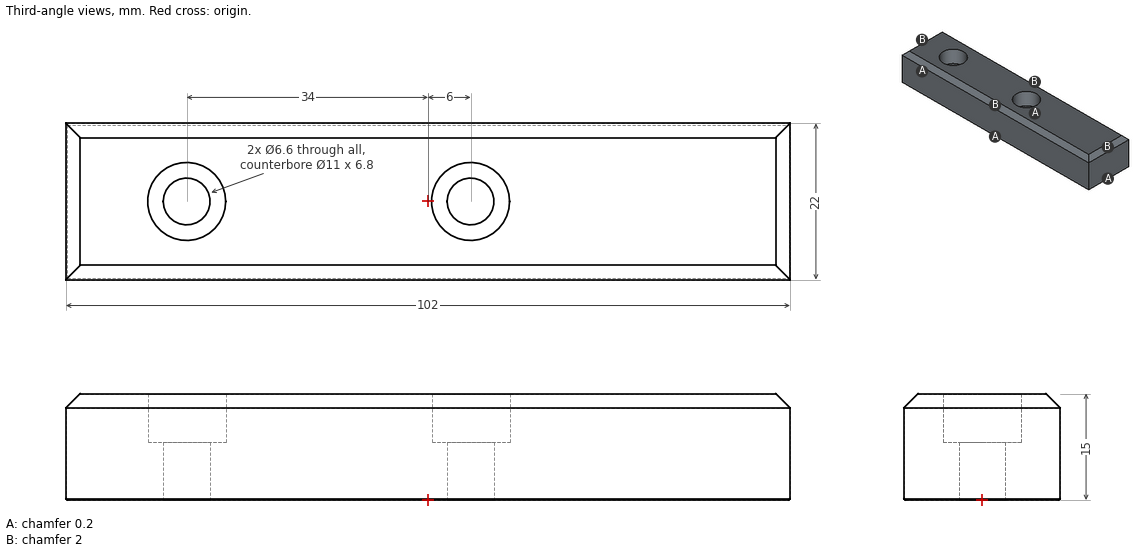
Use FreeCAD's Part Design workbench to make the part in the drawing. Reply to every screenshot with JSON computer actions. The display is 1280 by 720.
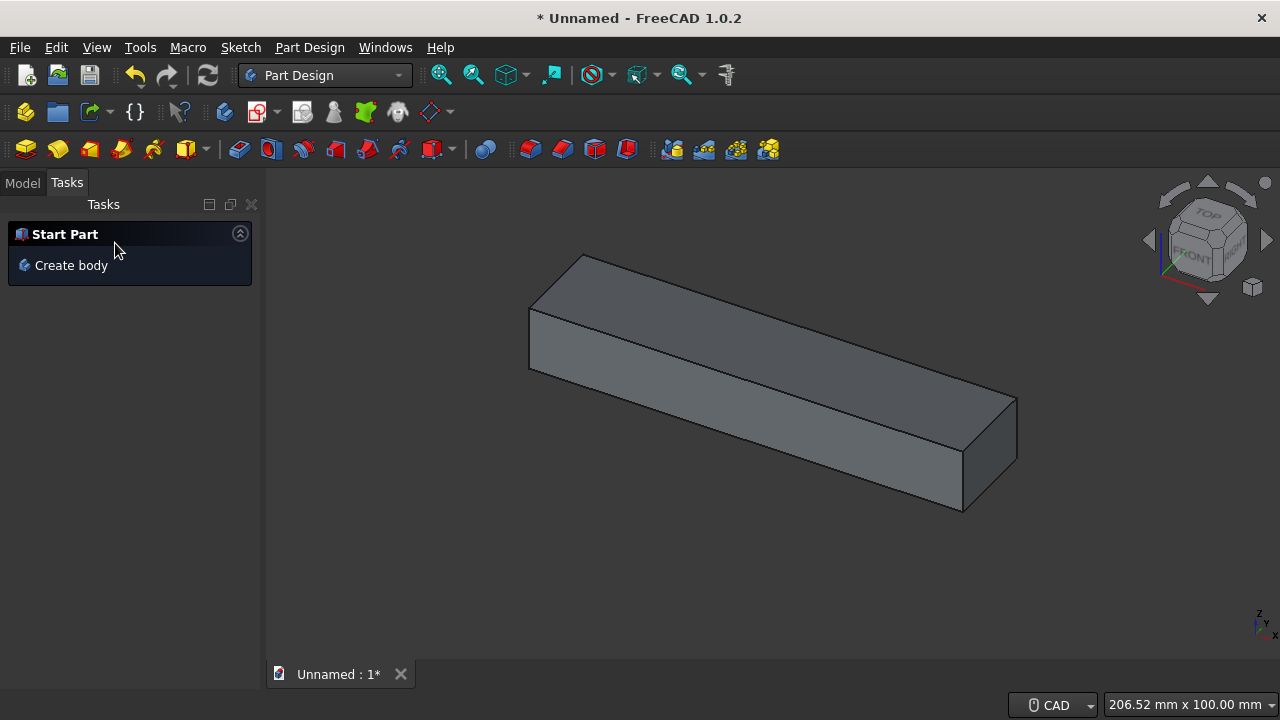
{"action": "left_click", "coordinate": [897, 393]}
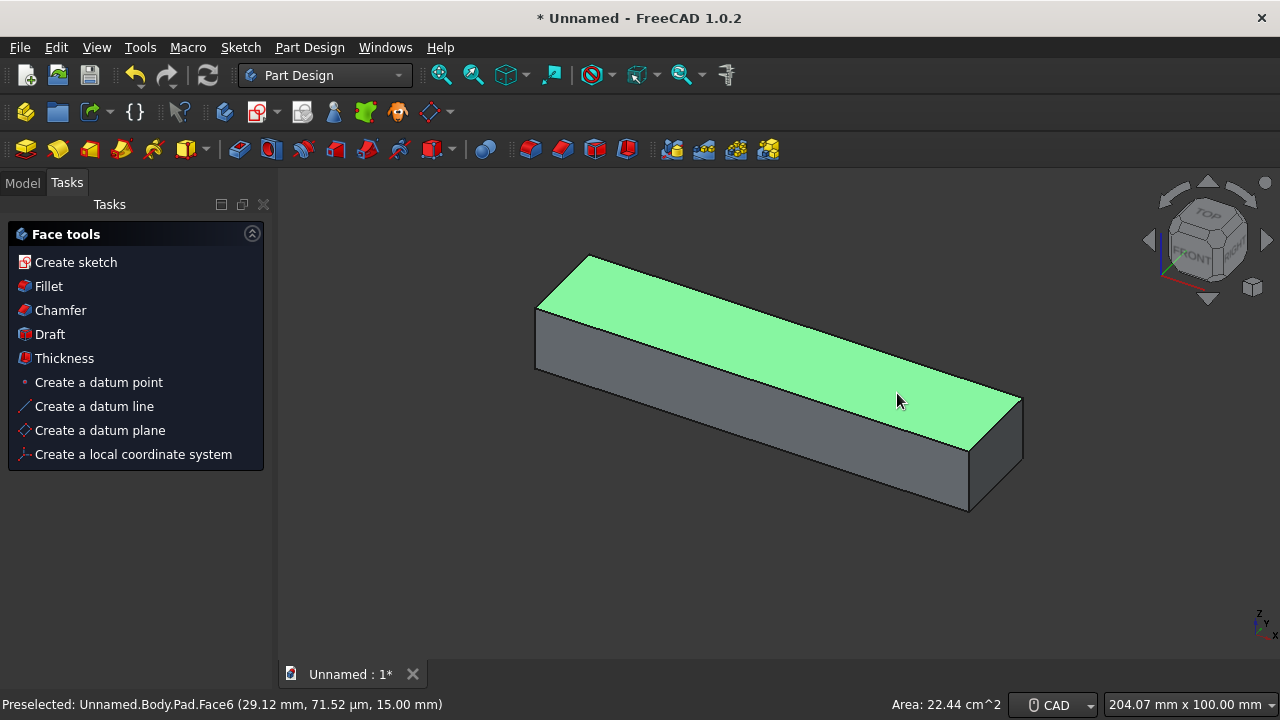
{"action": "left_click", "coordinate": [258, 112]}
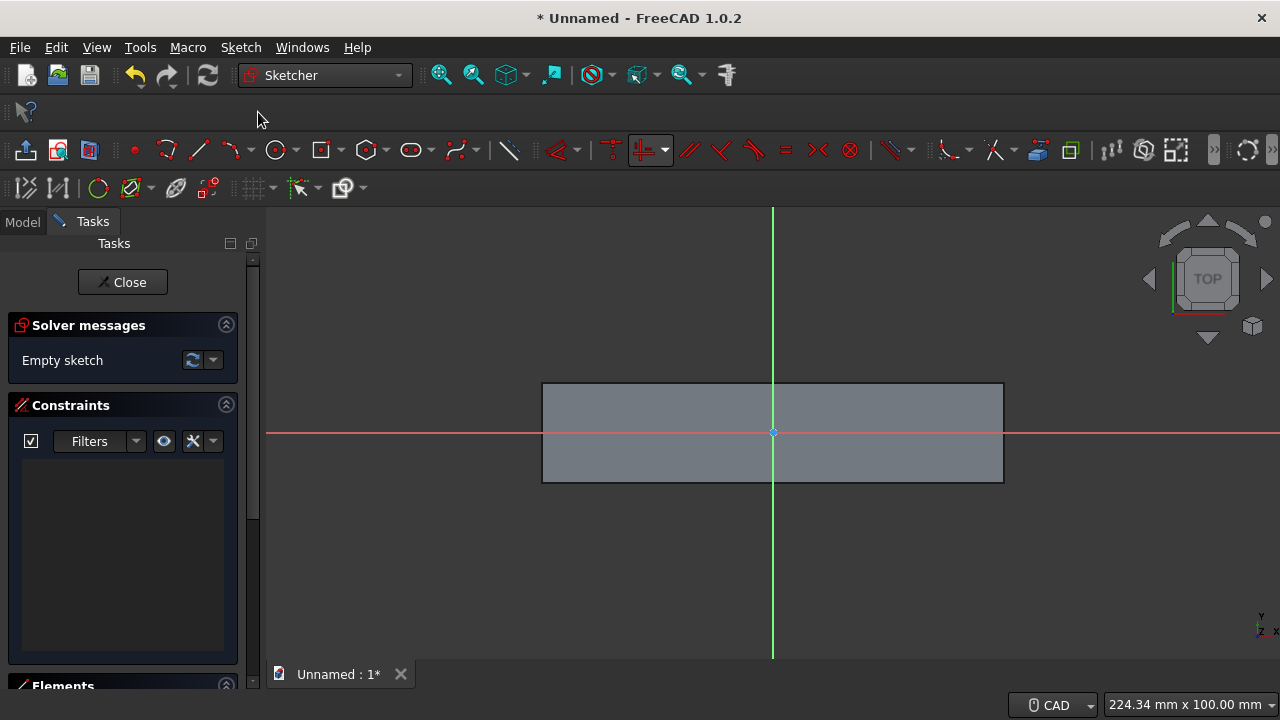
{"action": "scroll", "coordinate": [713, 433], "scroll_direction": "up", "scroll_amount": 5}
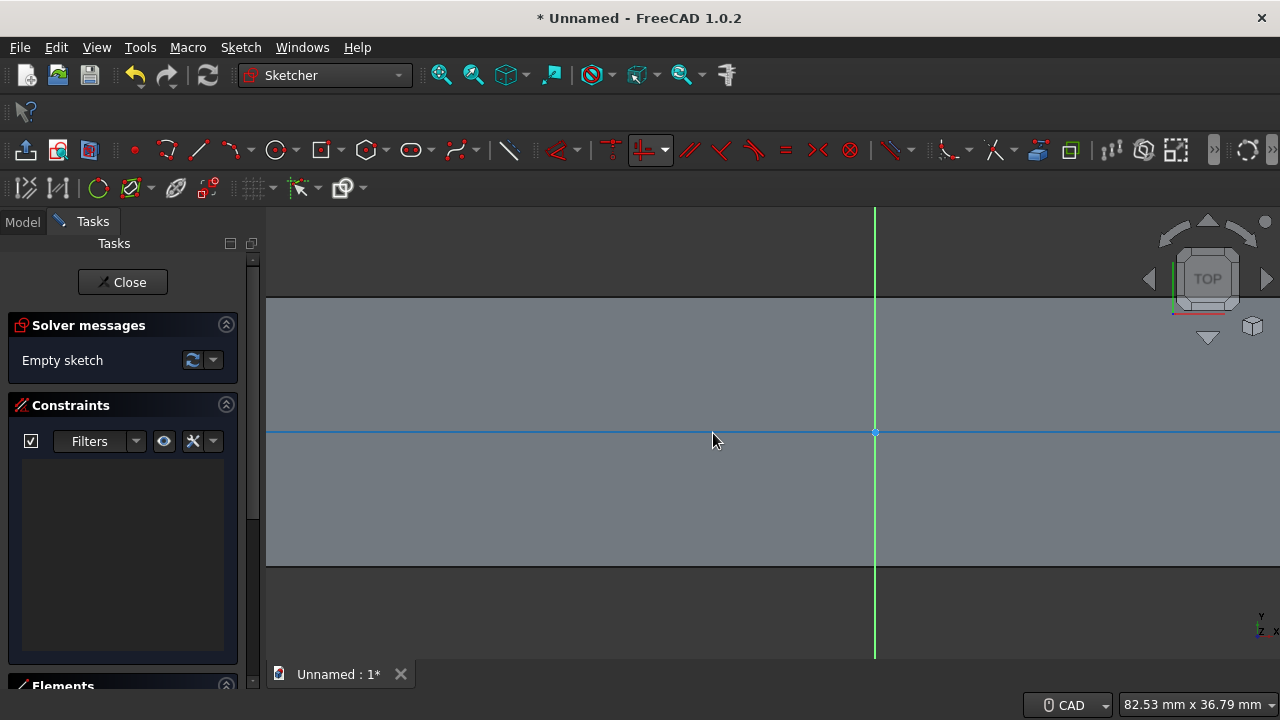
{"action": "left_click", "coordinate": [276, 150]}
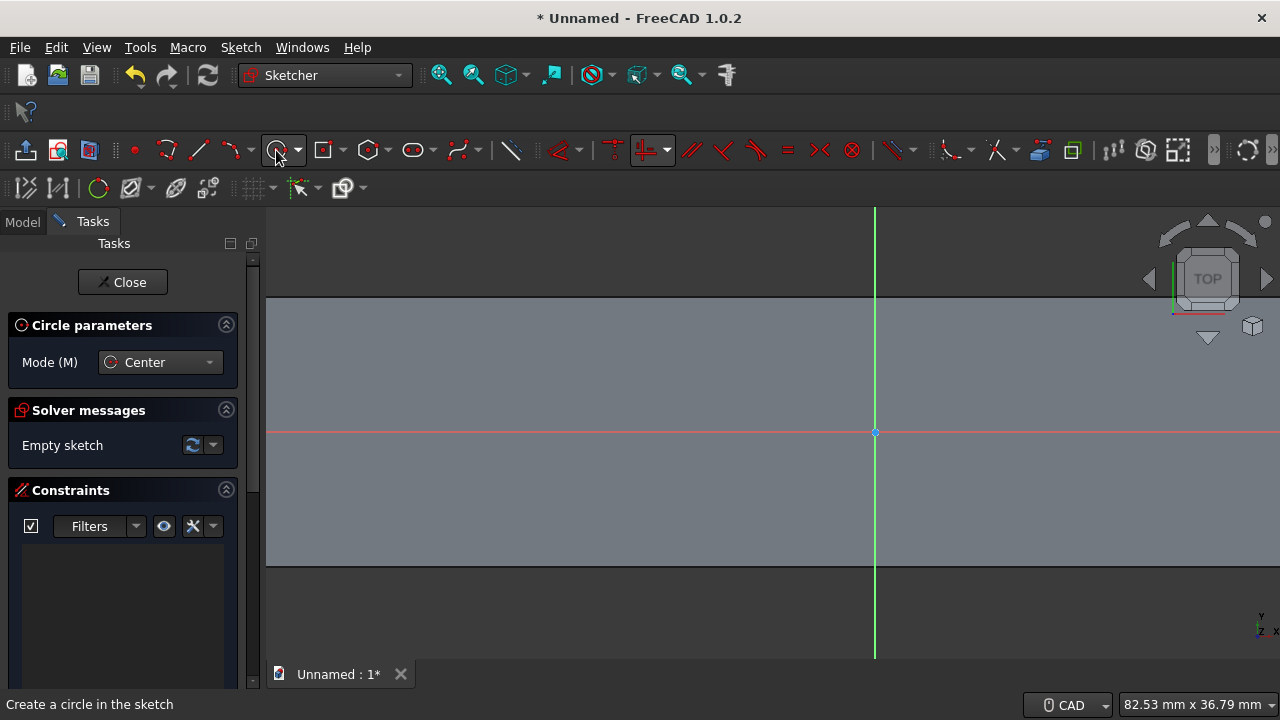
{"action": "left_click", "coordinate": [458, 432]}
{"action": "mouse_move", "coordinate": [486, 403]}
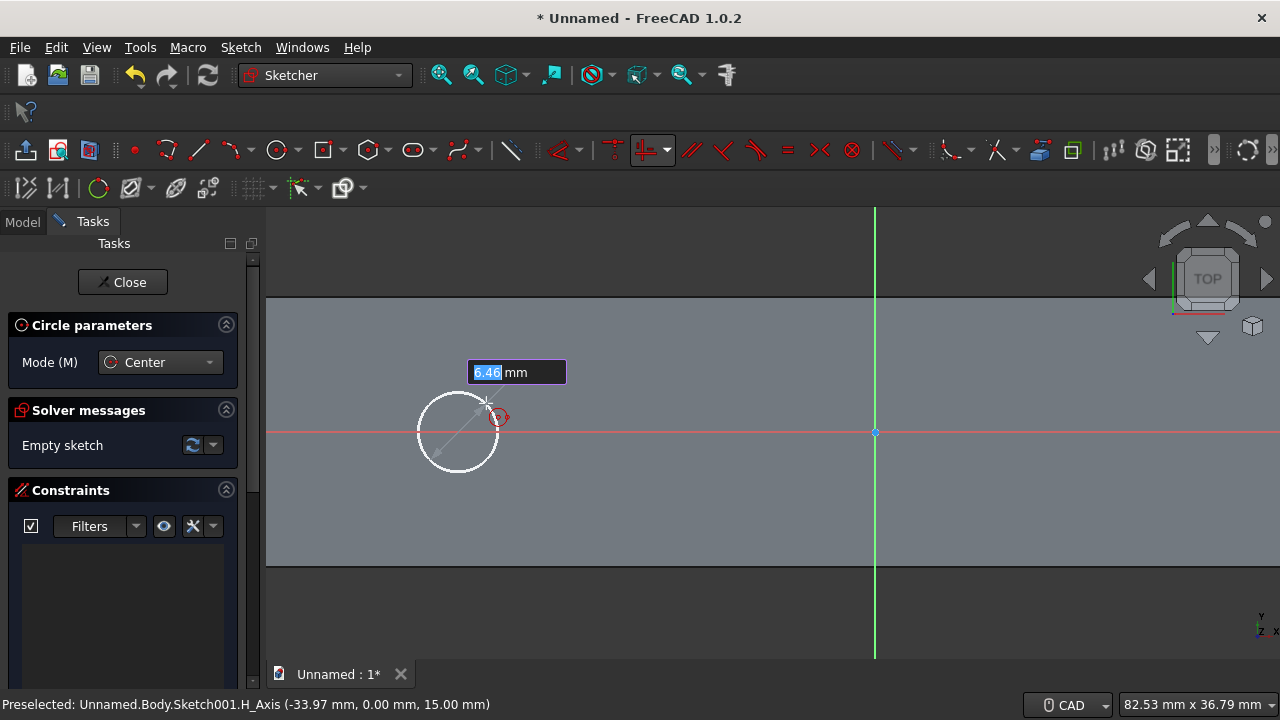
{"action": "type", "text": "6.6"}
{"action": "key", "text": "Return"}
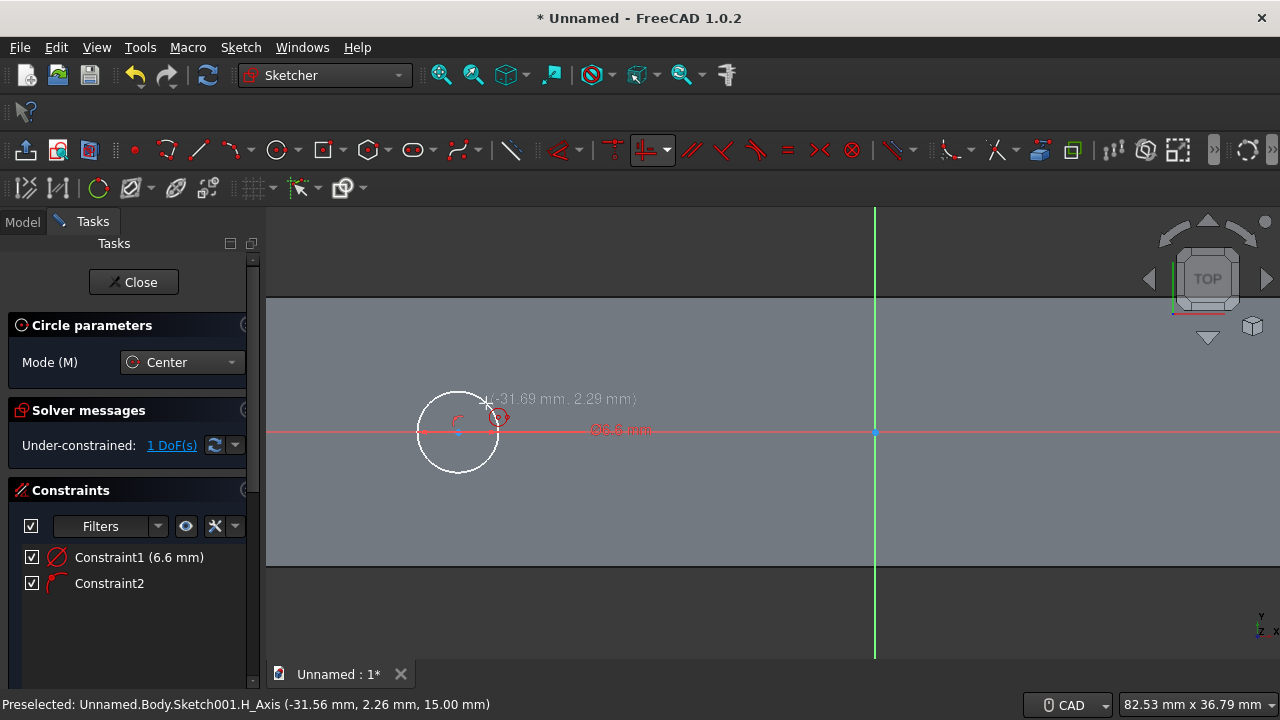
{"action": "left_click", "coordinate": [949, 432]}
{"action": "mouse_move", "coordinate": [978, 403]}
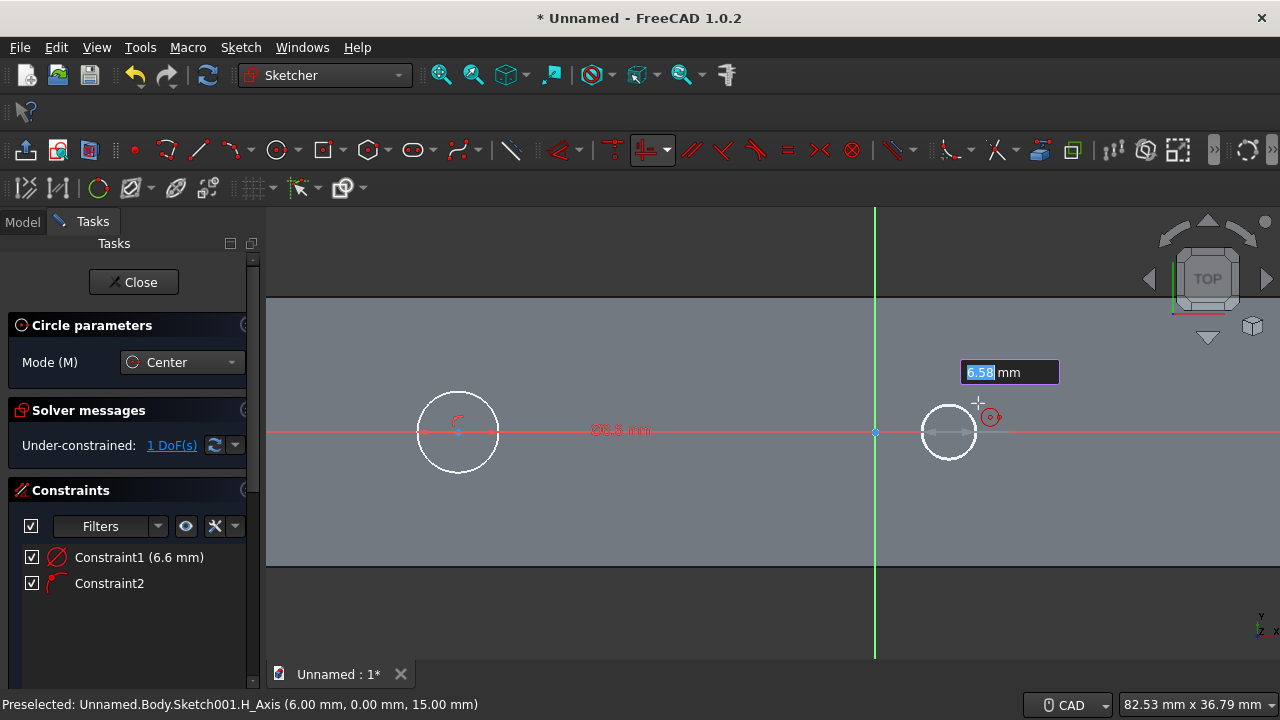
{"action": "type", "text": "6.6"}
{"action": "key", "text": "Return"}
{"action": "key", "text": "Escape"}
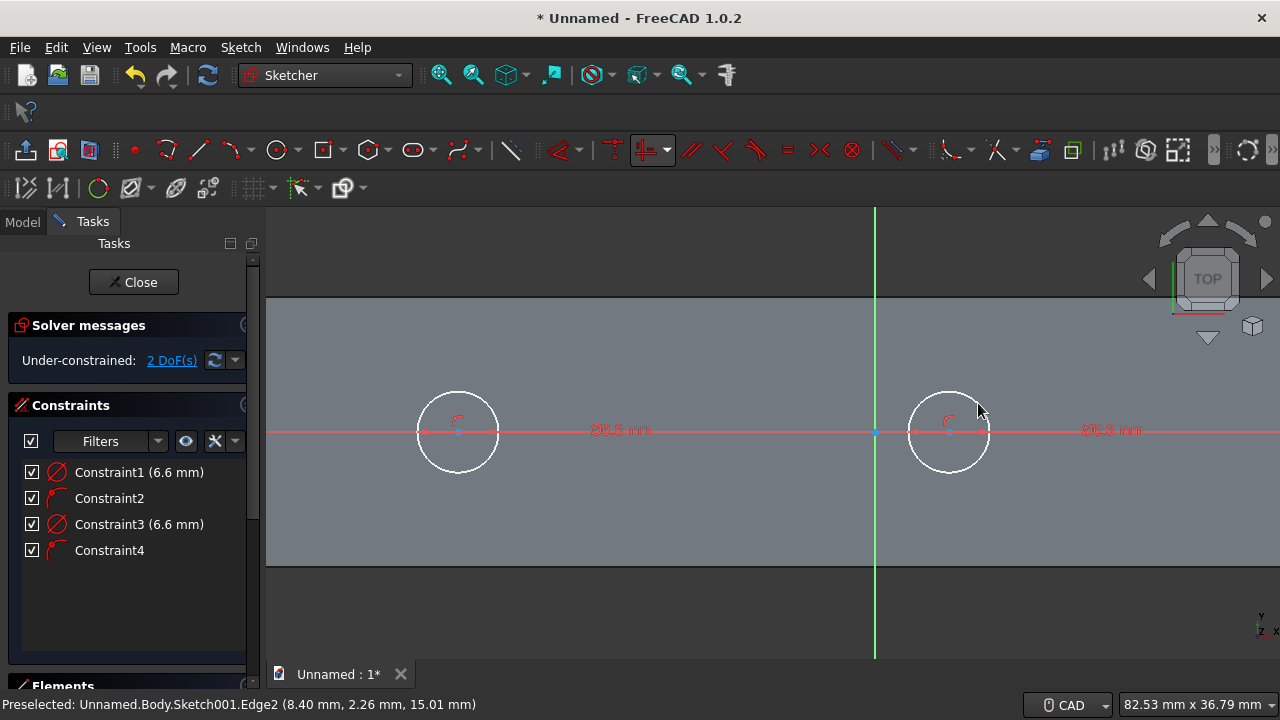
{"action": "left_click", "coordinate": [558, 150]}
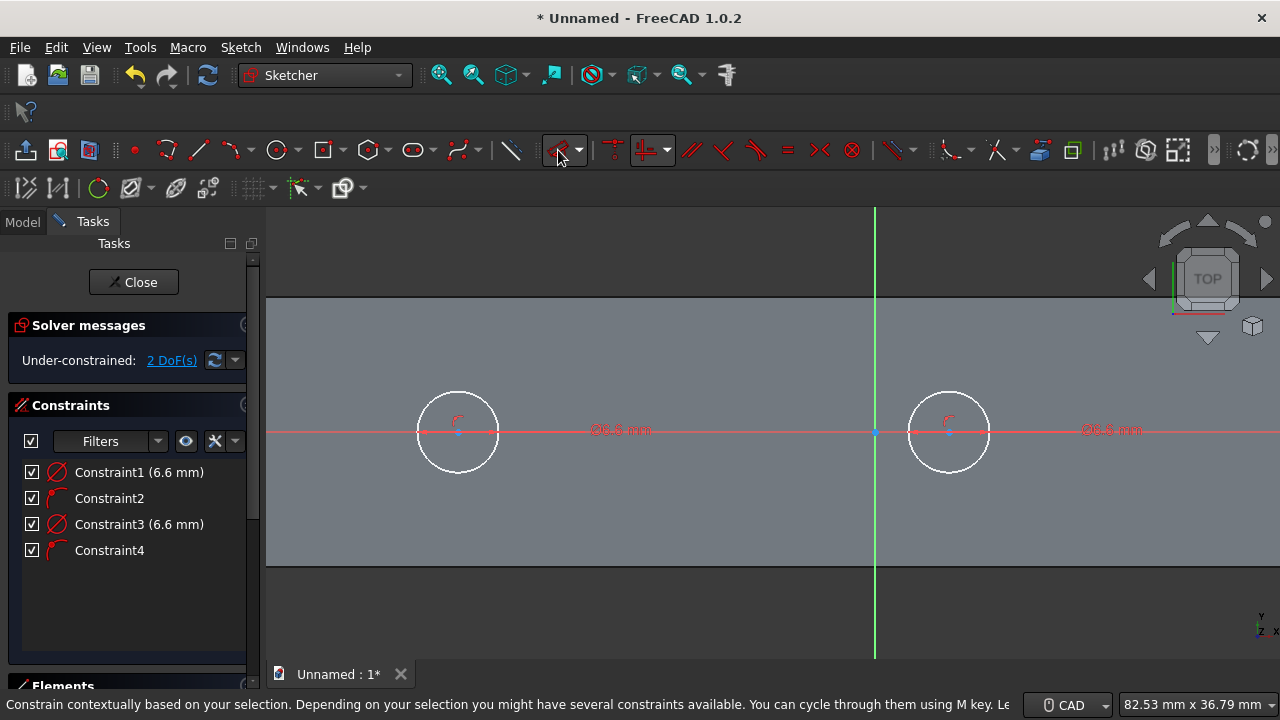
{"action": "left_click", "coordinate": [949, 432]}
{"action": "left_click", "coordinate": [895, 466]}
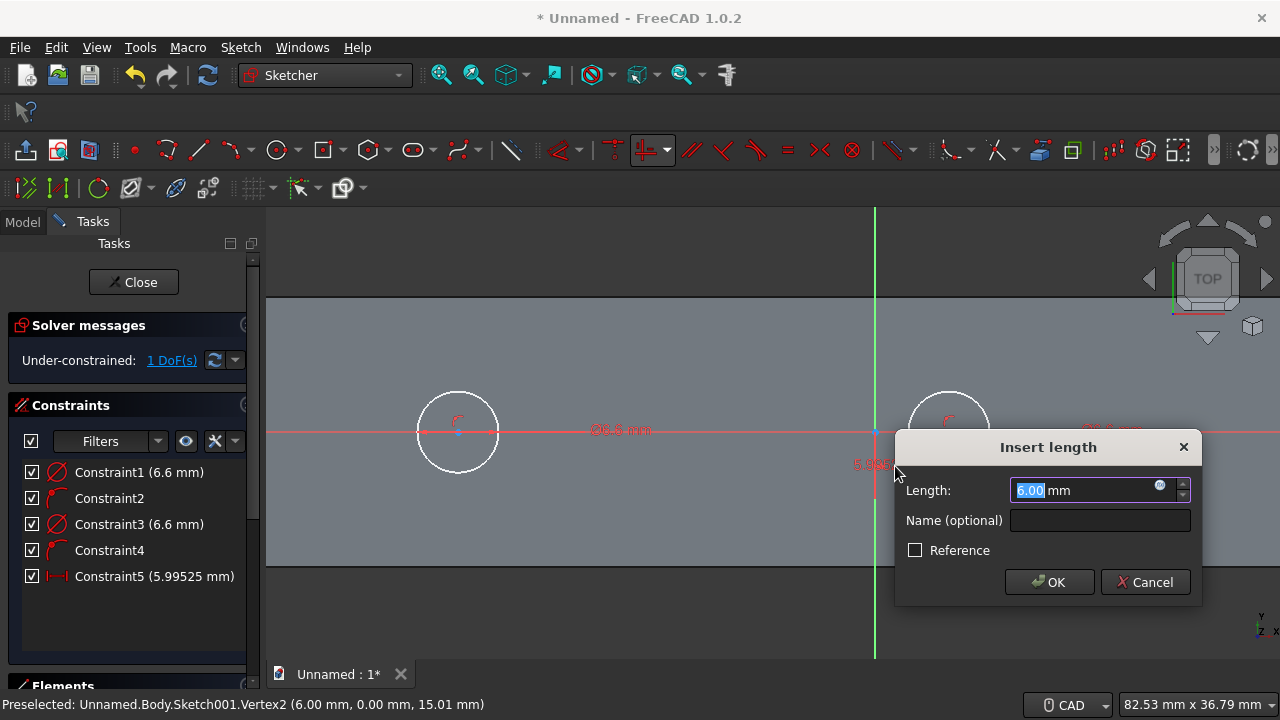
{"action": "type", "text": "6"}
{"action": "key", "text": "Return"}